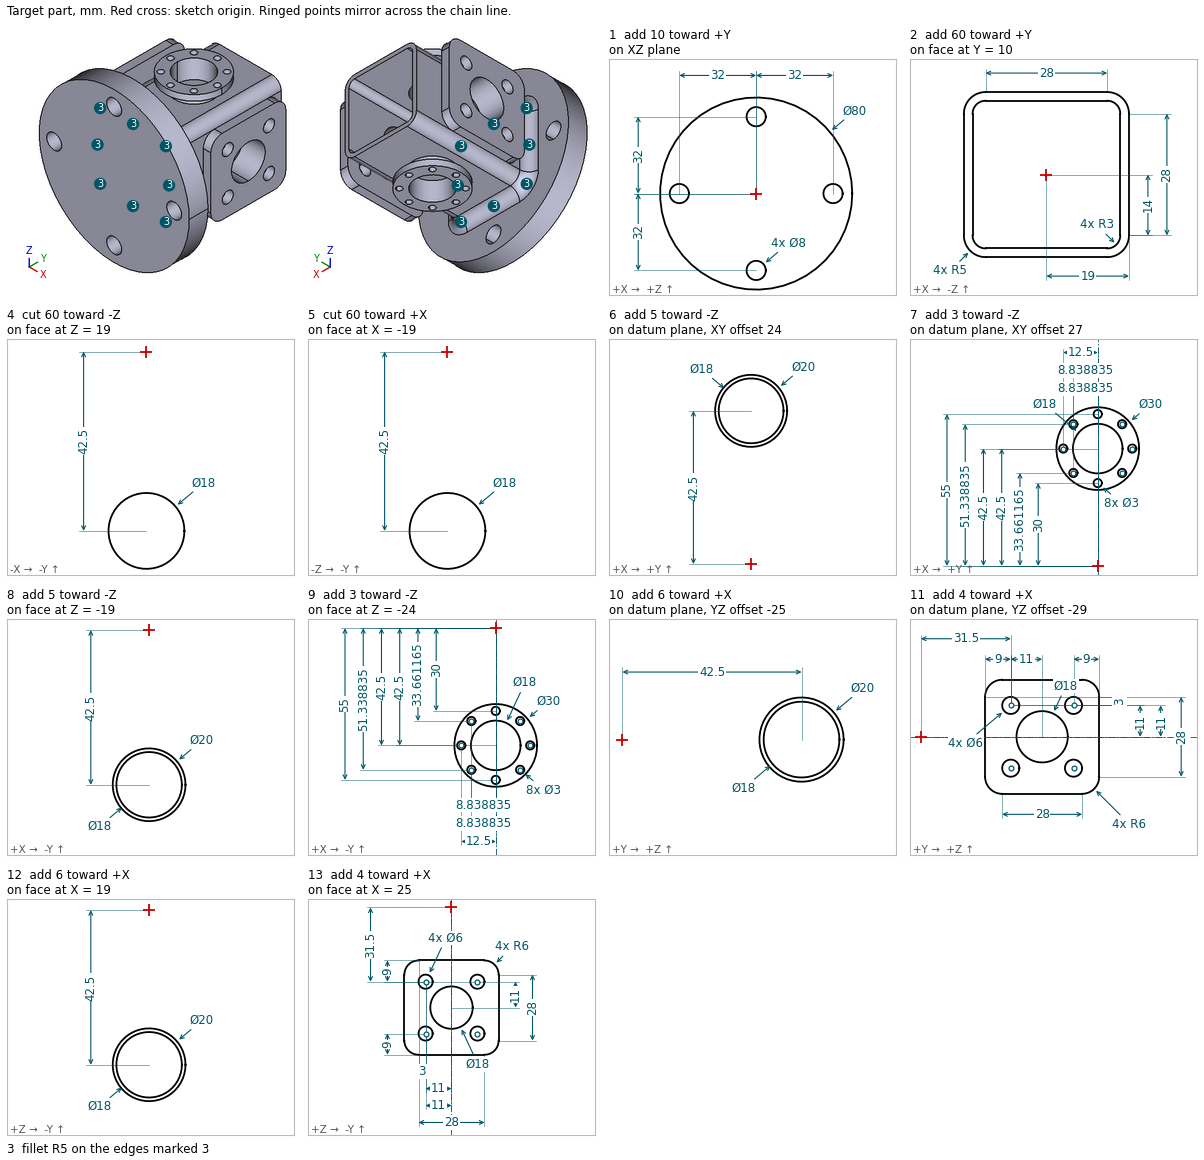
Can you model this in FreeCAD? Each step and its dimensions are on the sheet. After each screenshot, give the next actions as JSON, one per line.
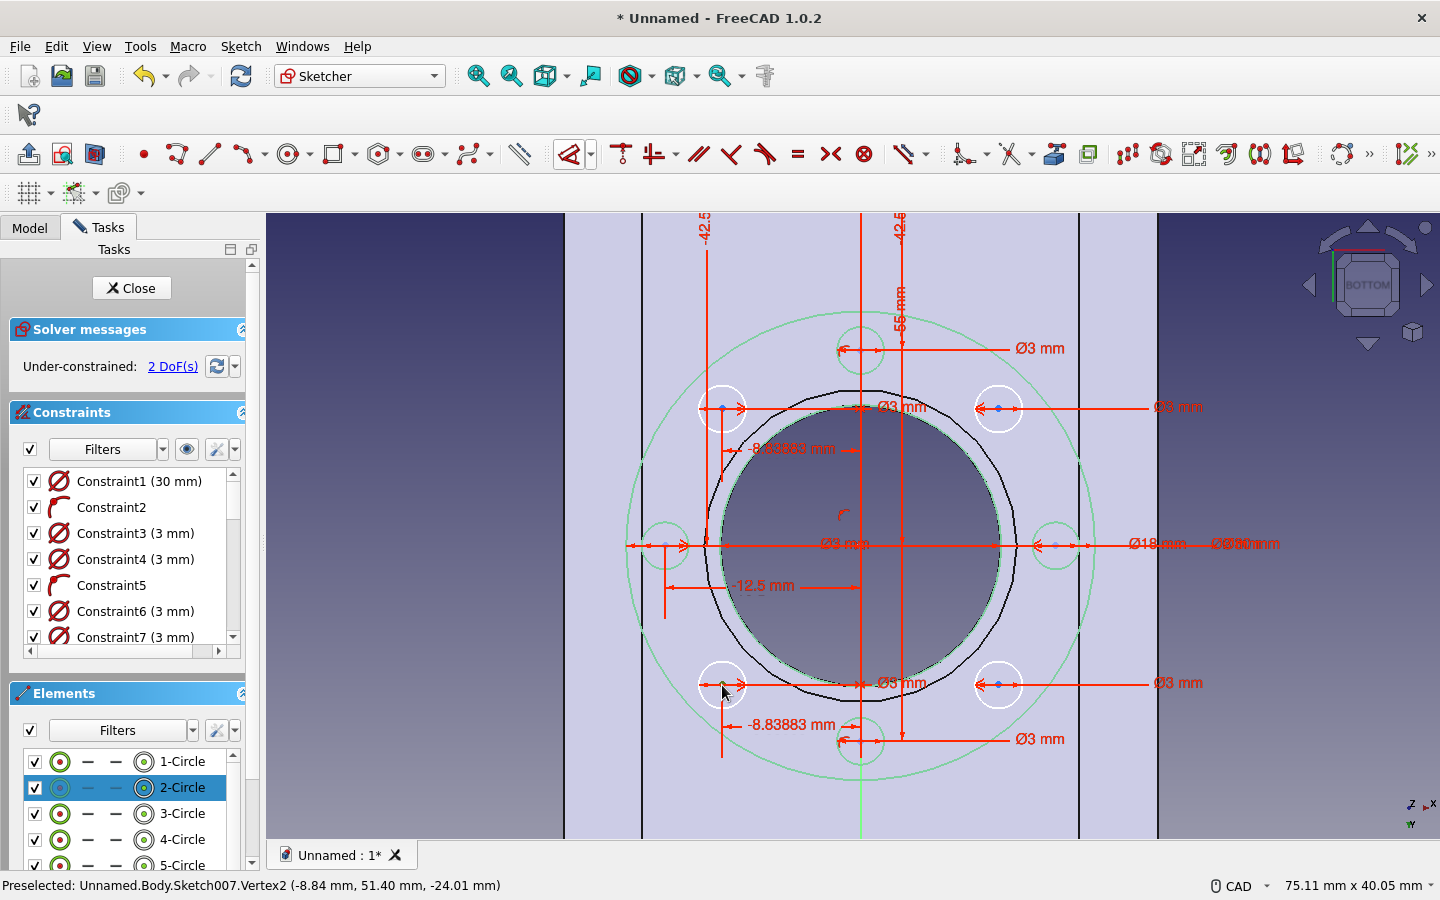
{"action": "key", "text": "i"}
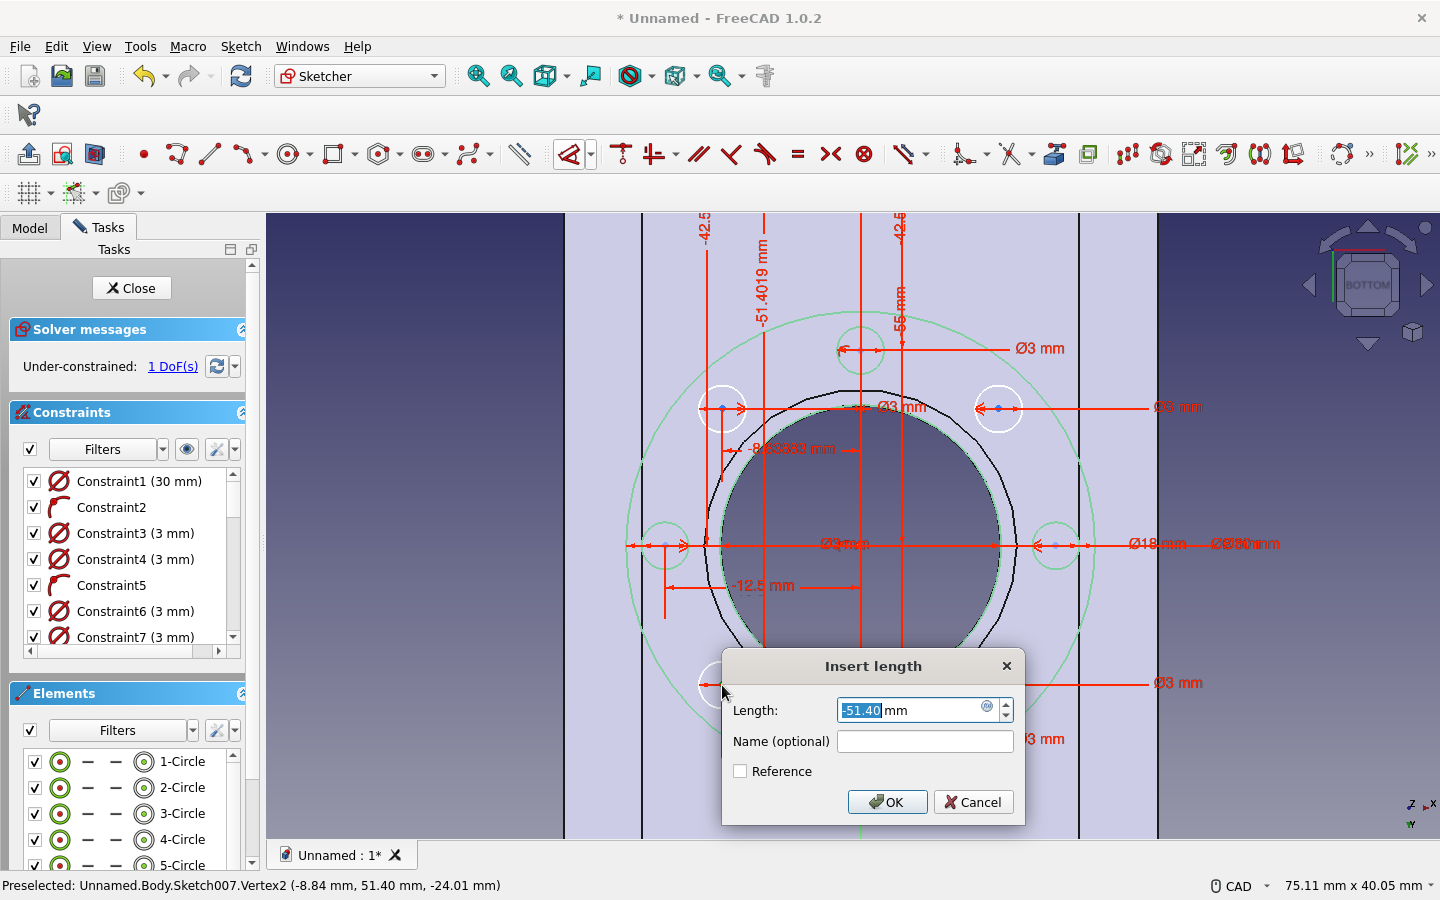
{"action": "type", "text": "-51.338835"}
{"action": "key", "text": "Return"}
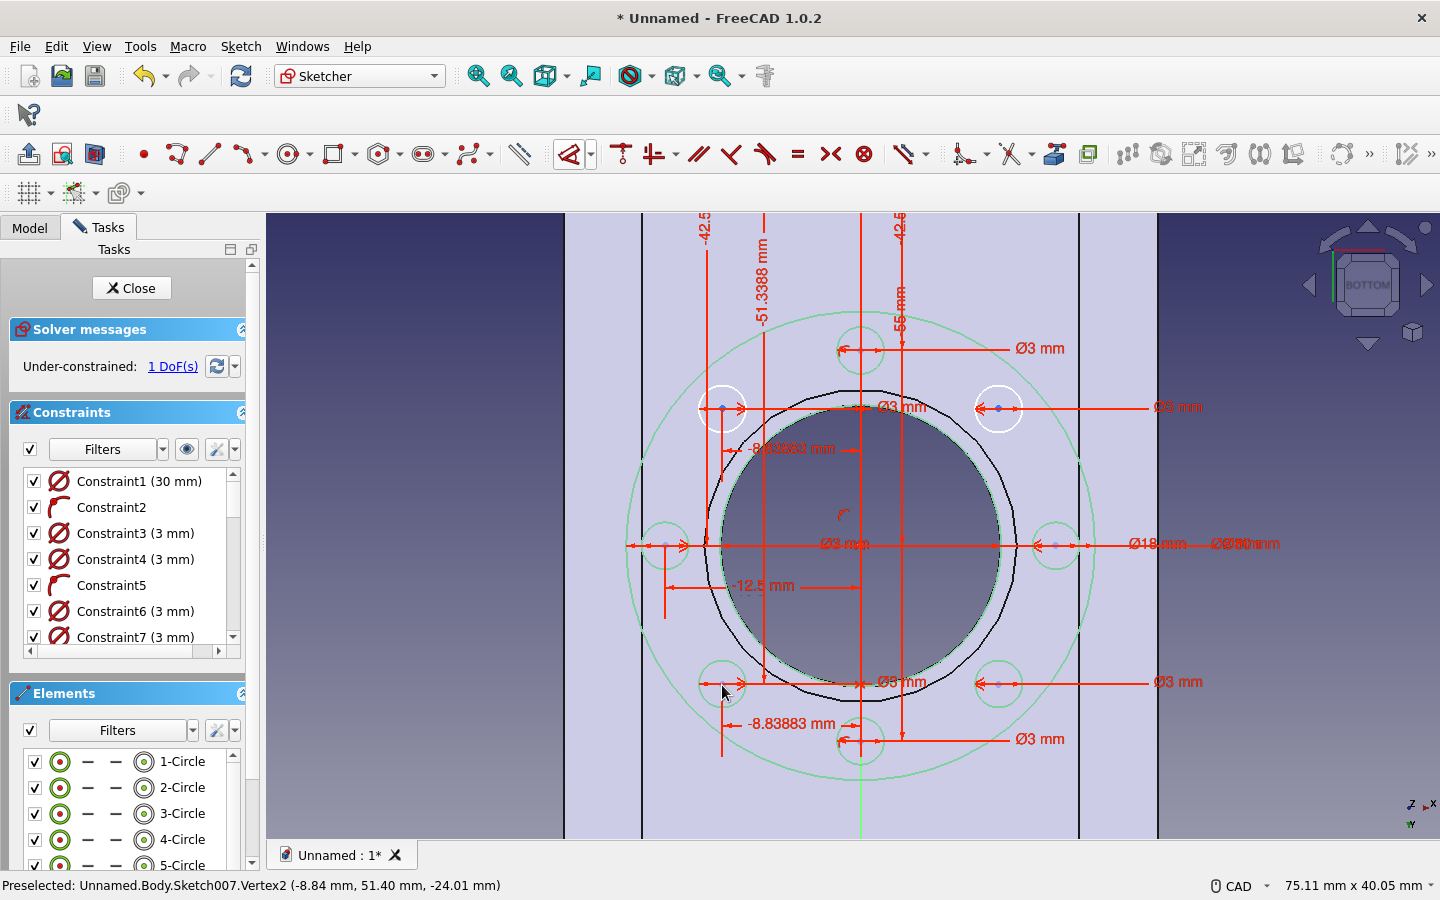
{"action": "left_click", "coordinate": [722, 409]}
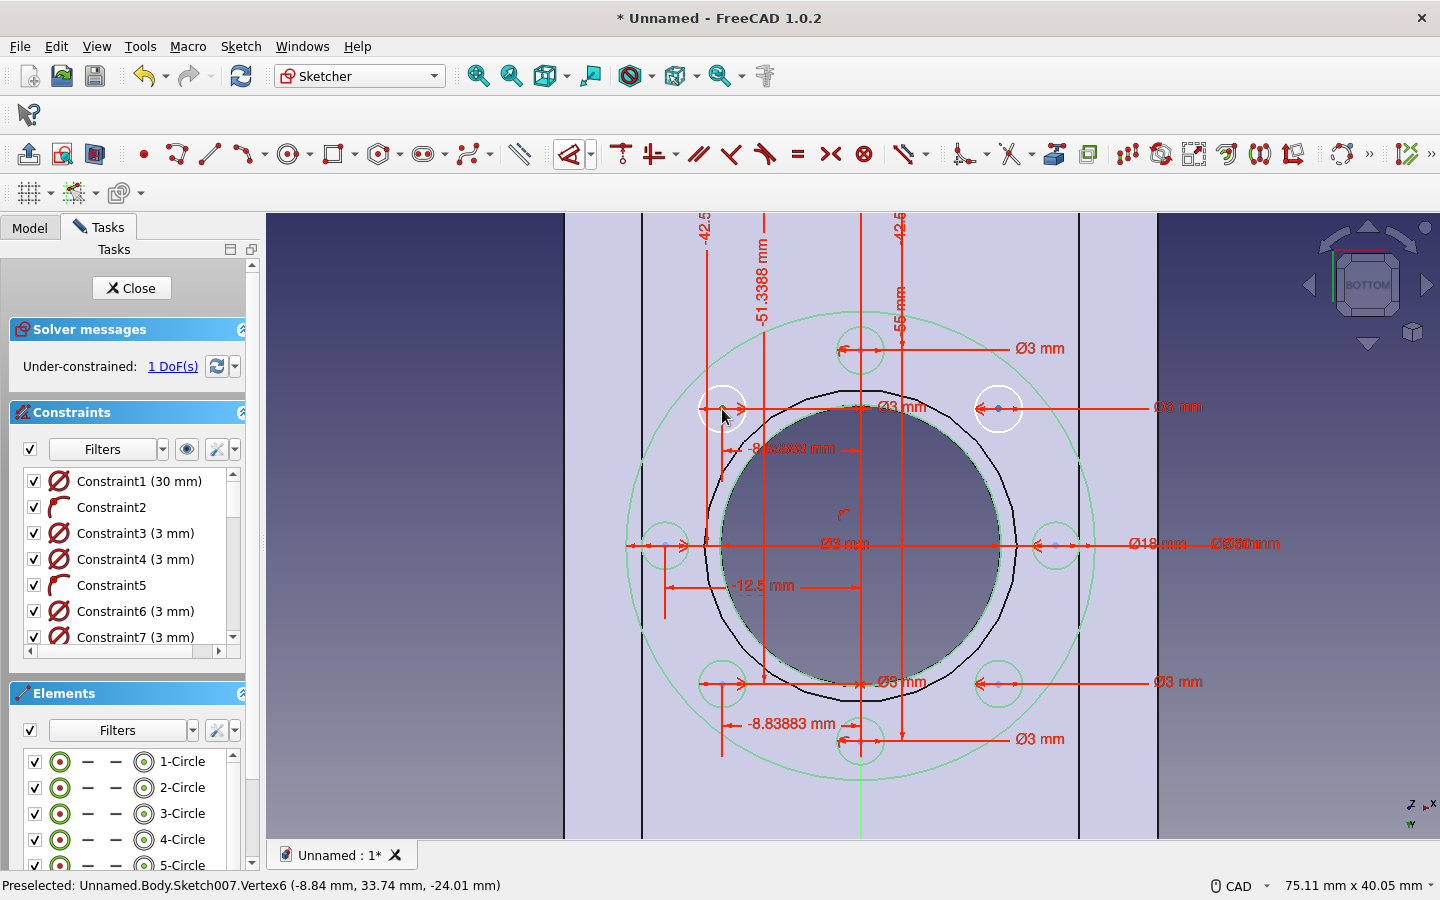
{"action": "key", "text": "i"}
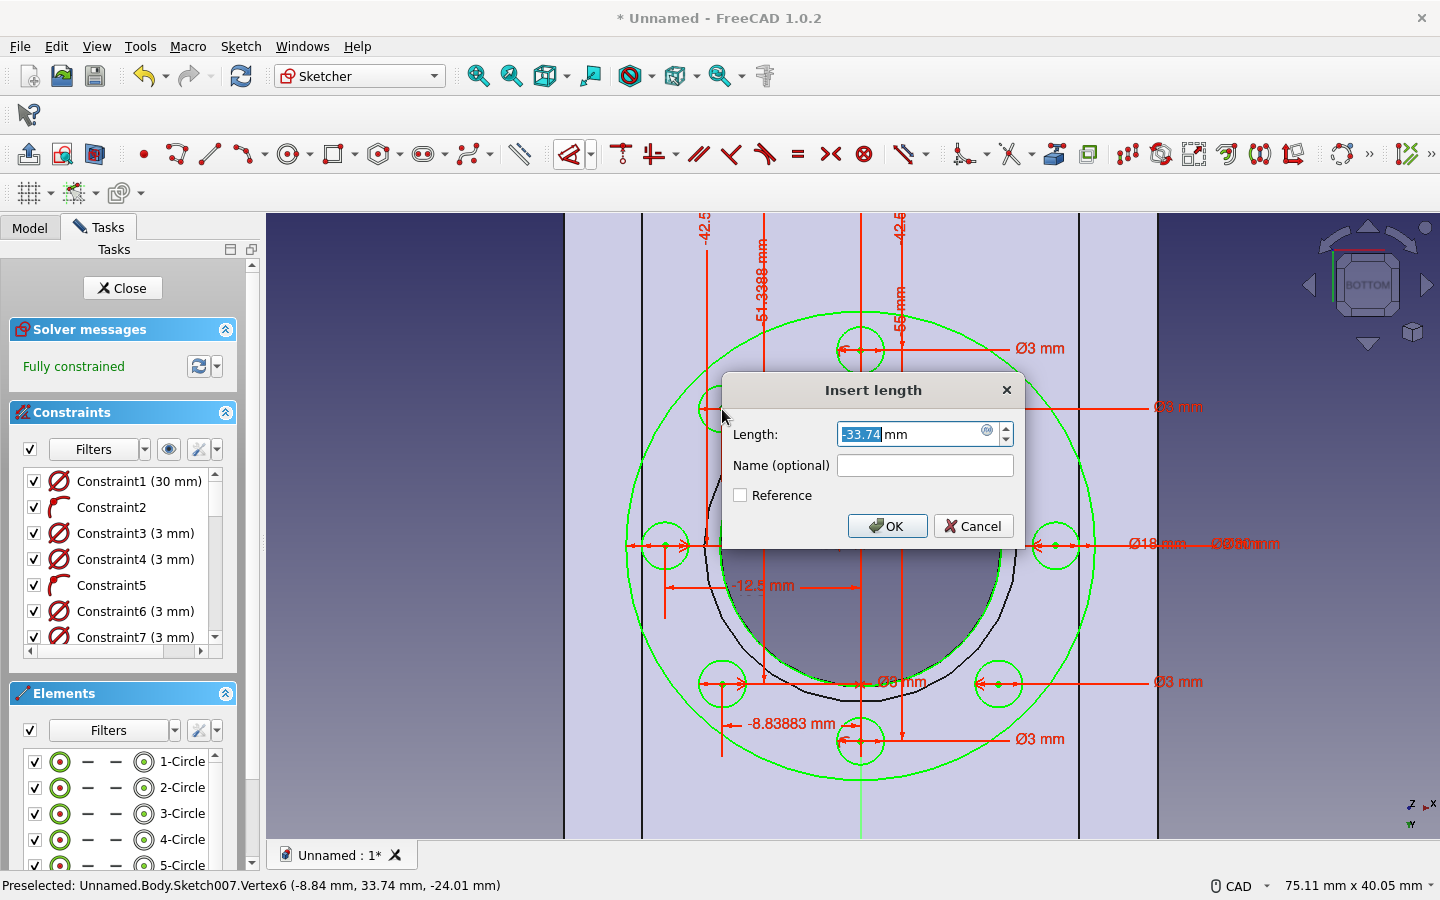
{"action": "type", "text": "-33.661165"}
{"action": "key", "text": "Return"}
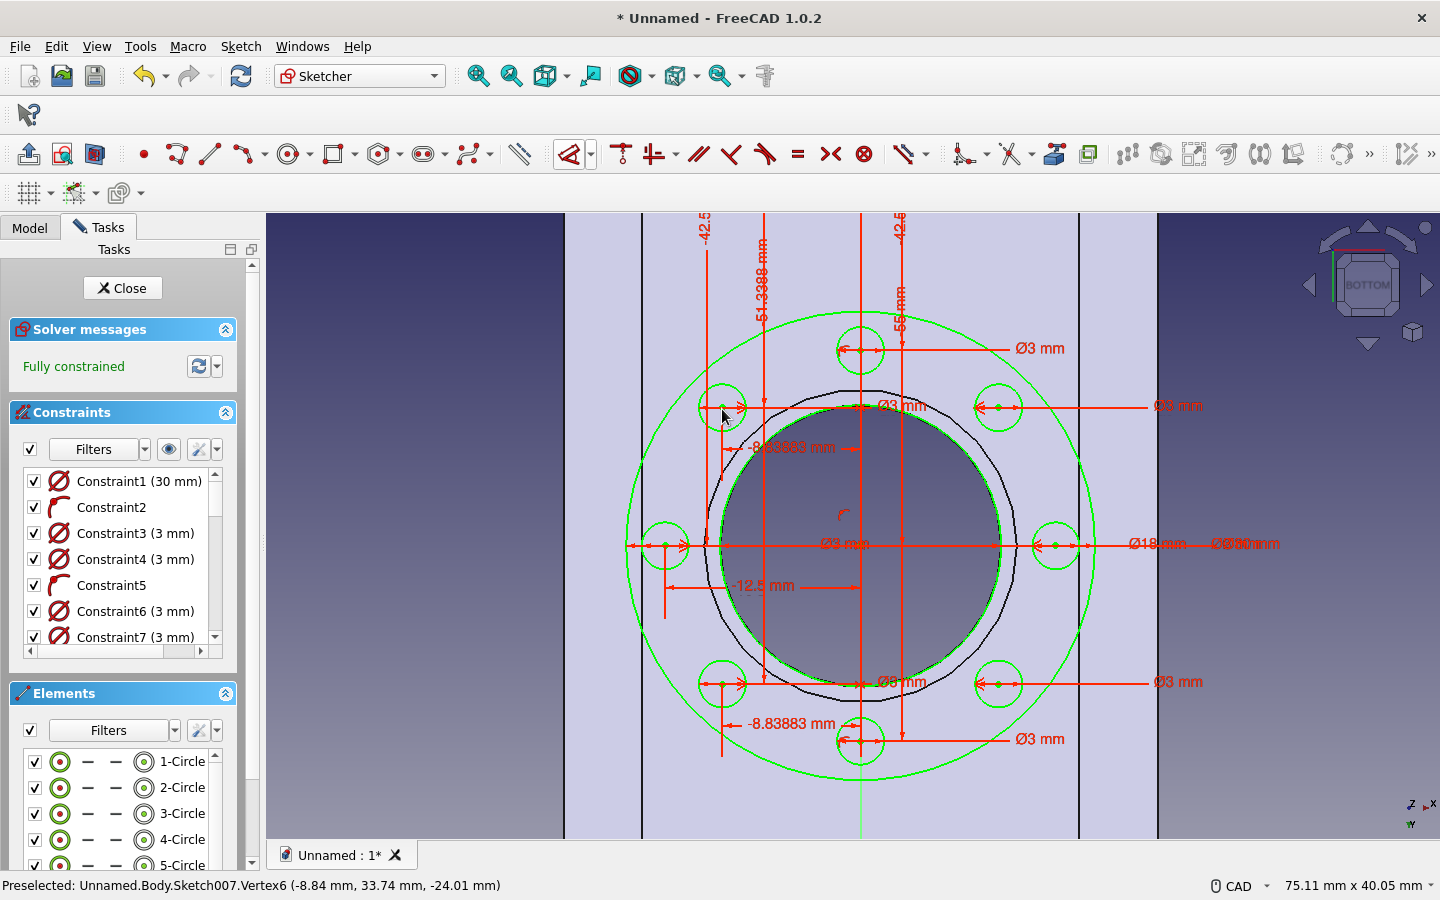
{"action": "left_click", "coordinate": [123, 288]}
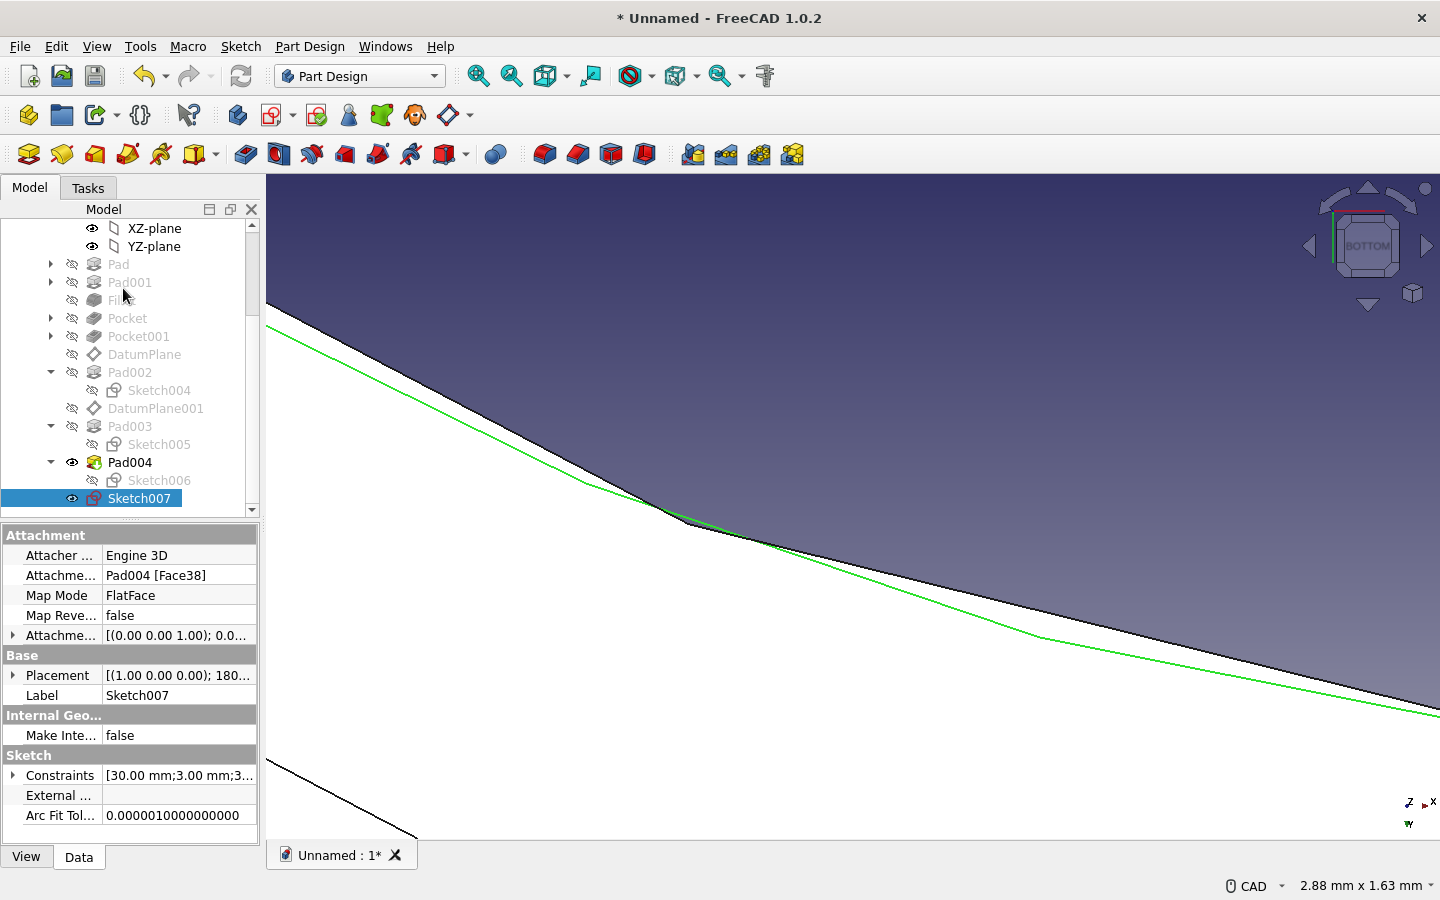
{"action": "left_click", "coordinate": [29, 154]}